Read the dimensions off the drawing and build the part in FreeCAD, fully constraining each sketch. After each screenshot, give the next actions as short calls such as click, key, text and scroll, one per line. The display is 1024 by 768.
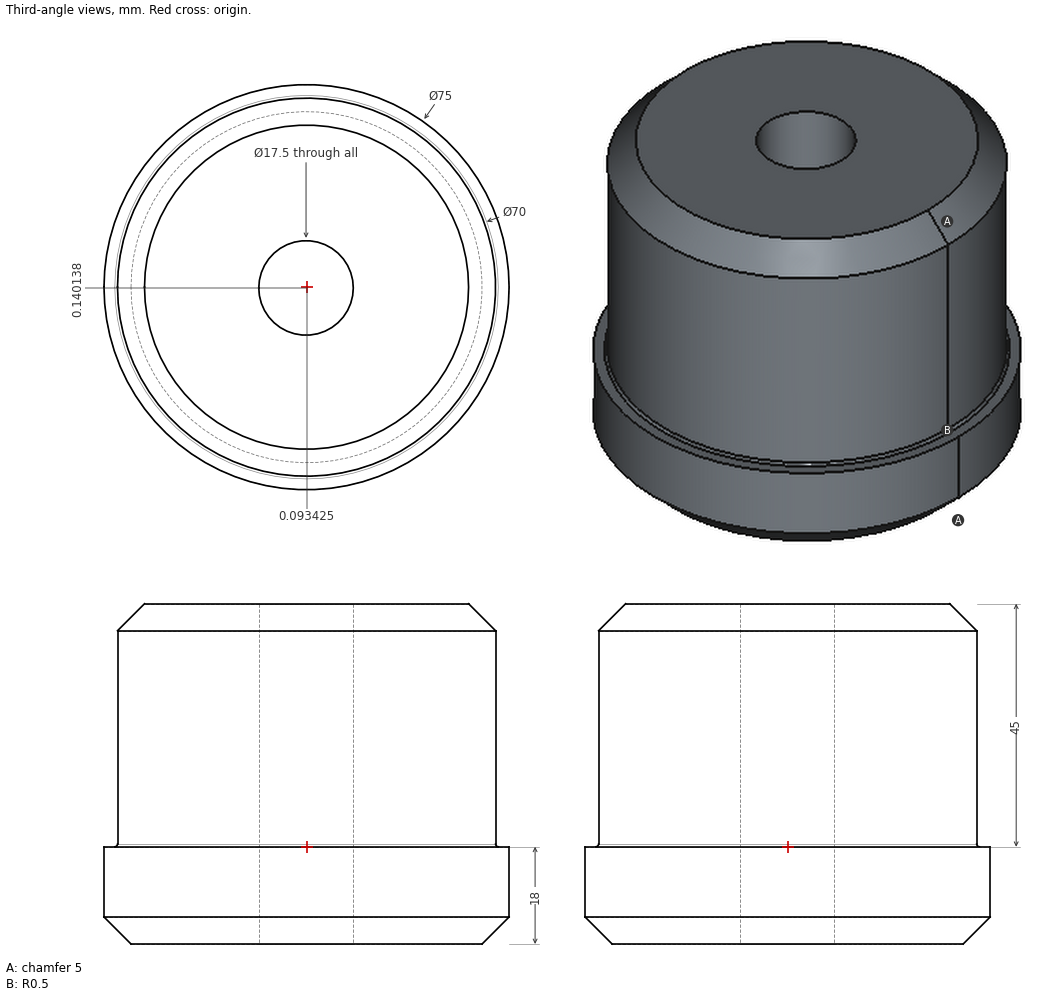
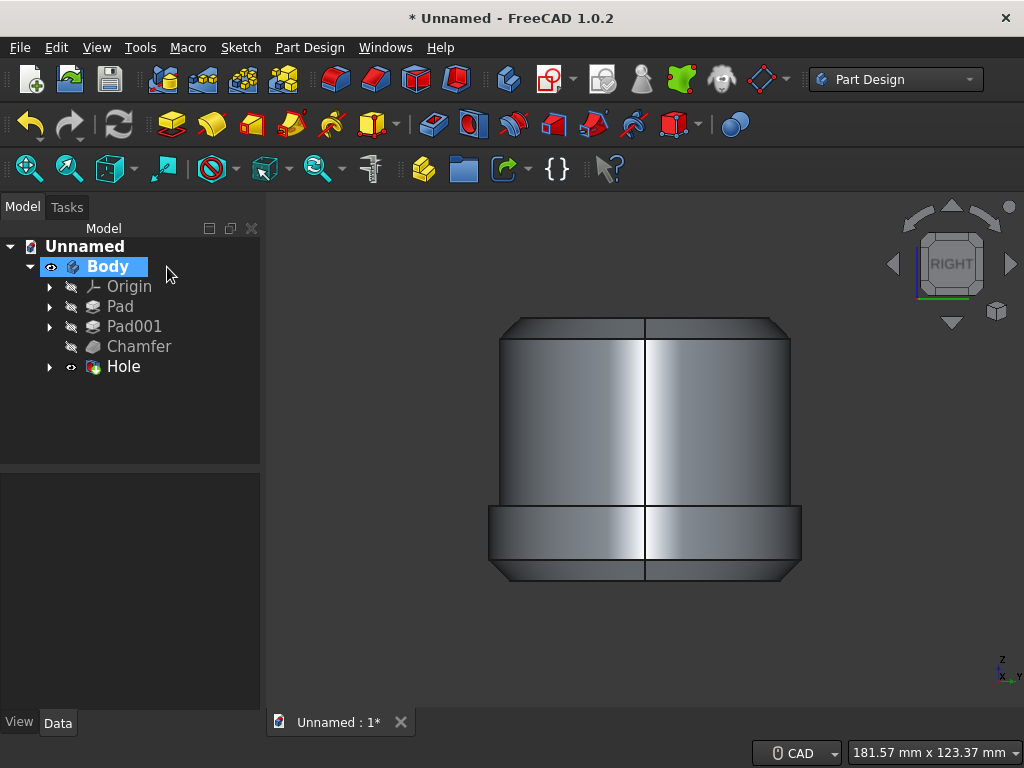
key(5)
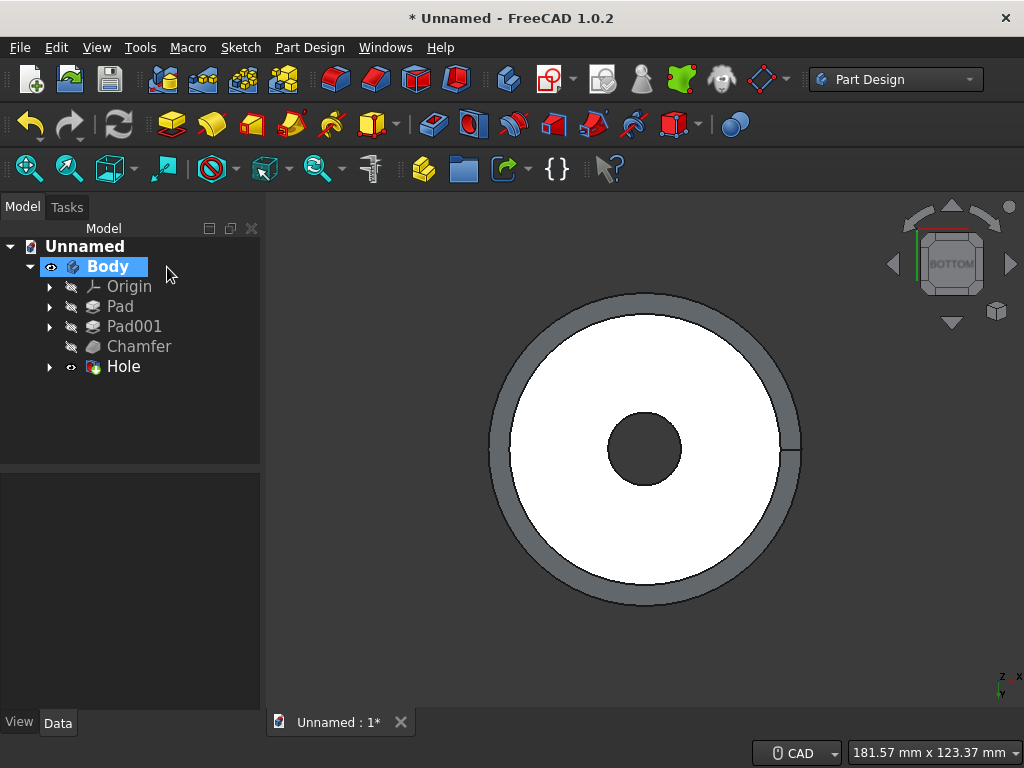
key(4)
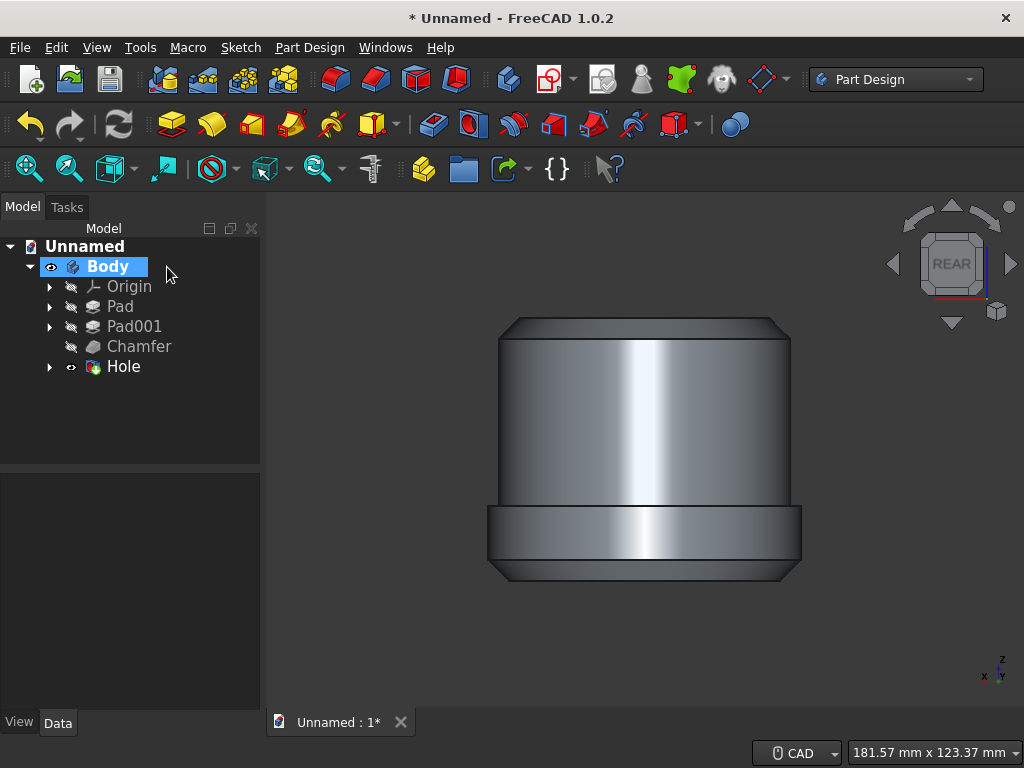
key(6)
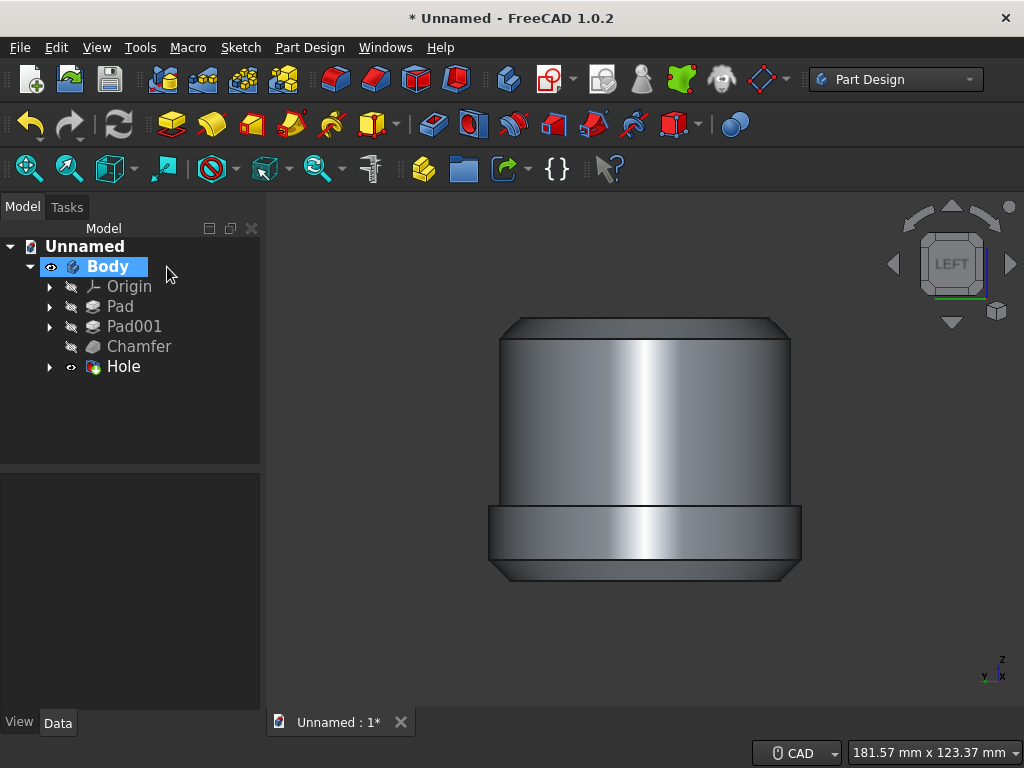
key(v)
key(3)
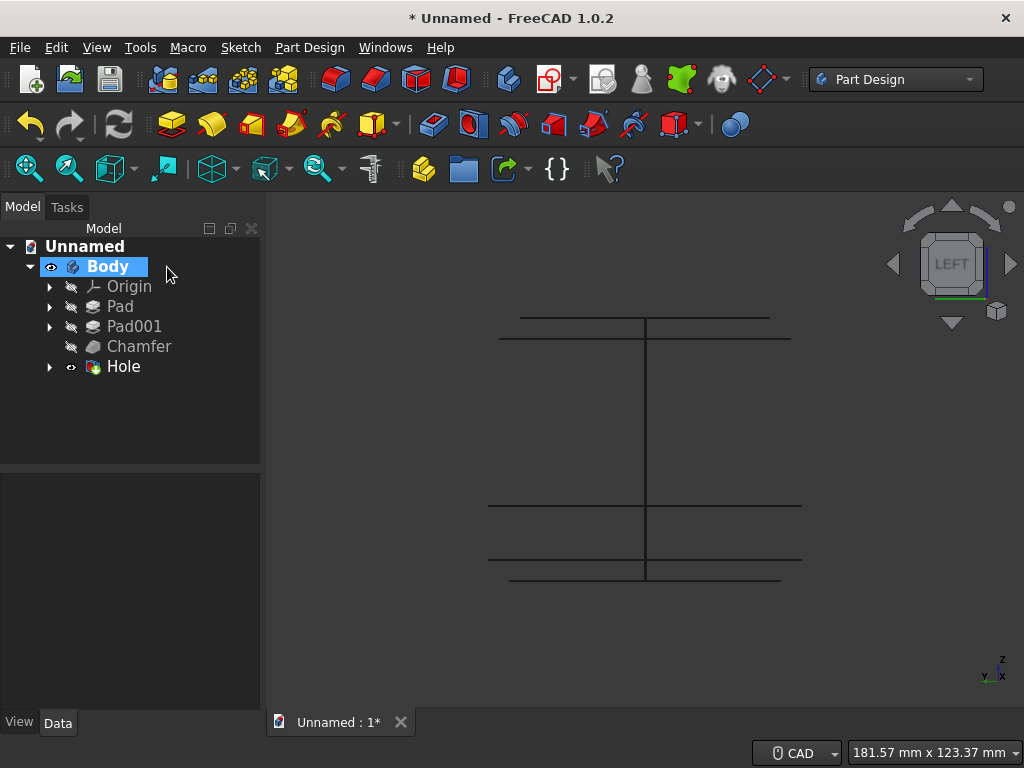
key(0)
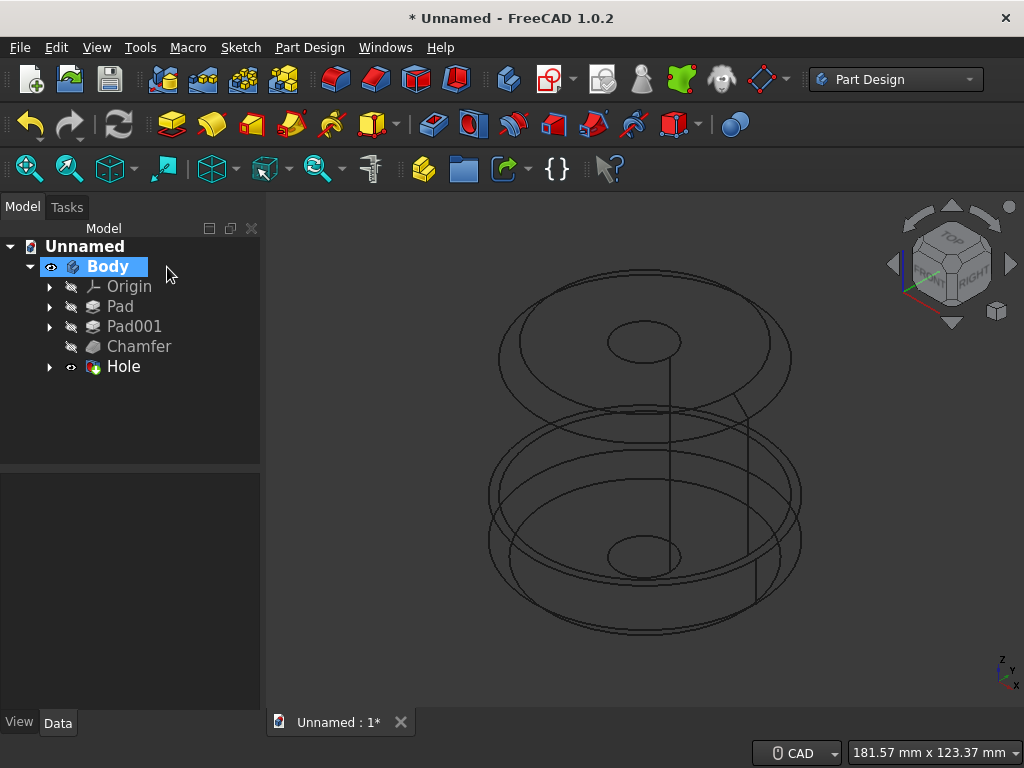
click(542, 435)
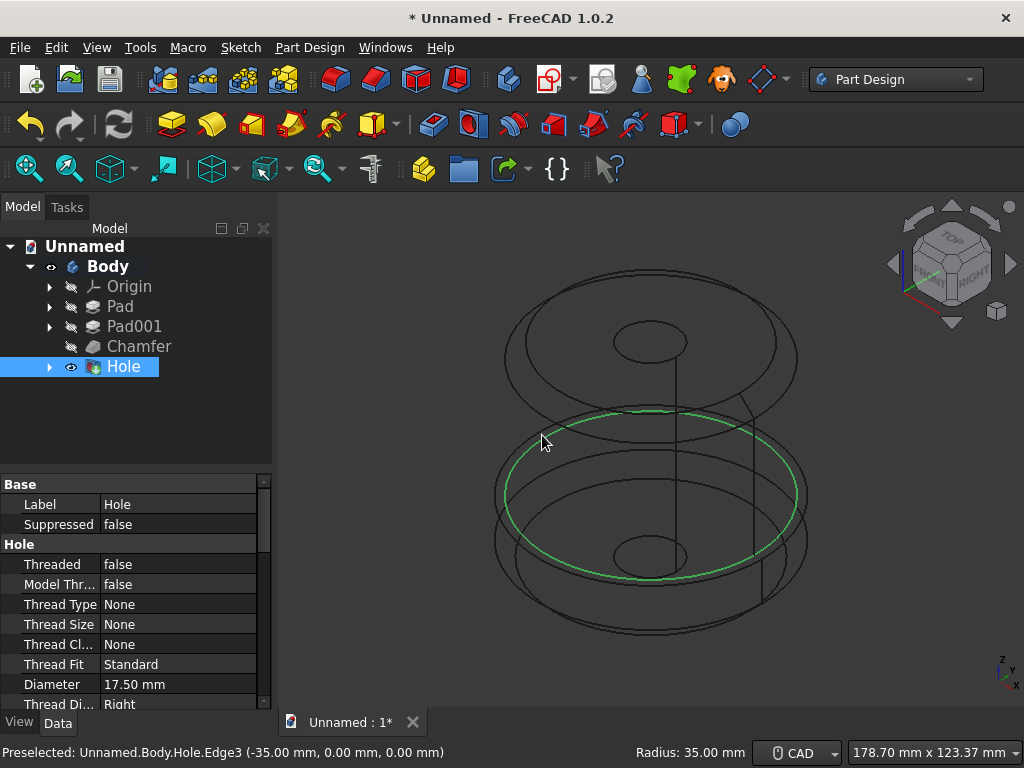
key(v)
key(1)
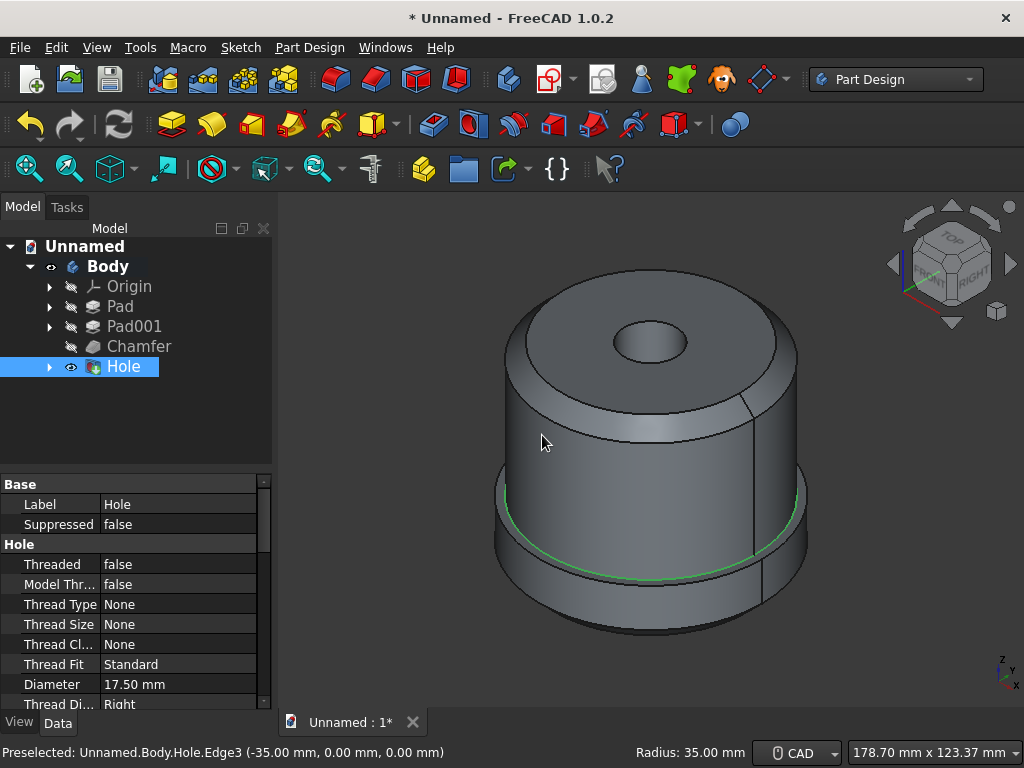
click(336, 80)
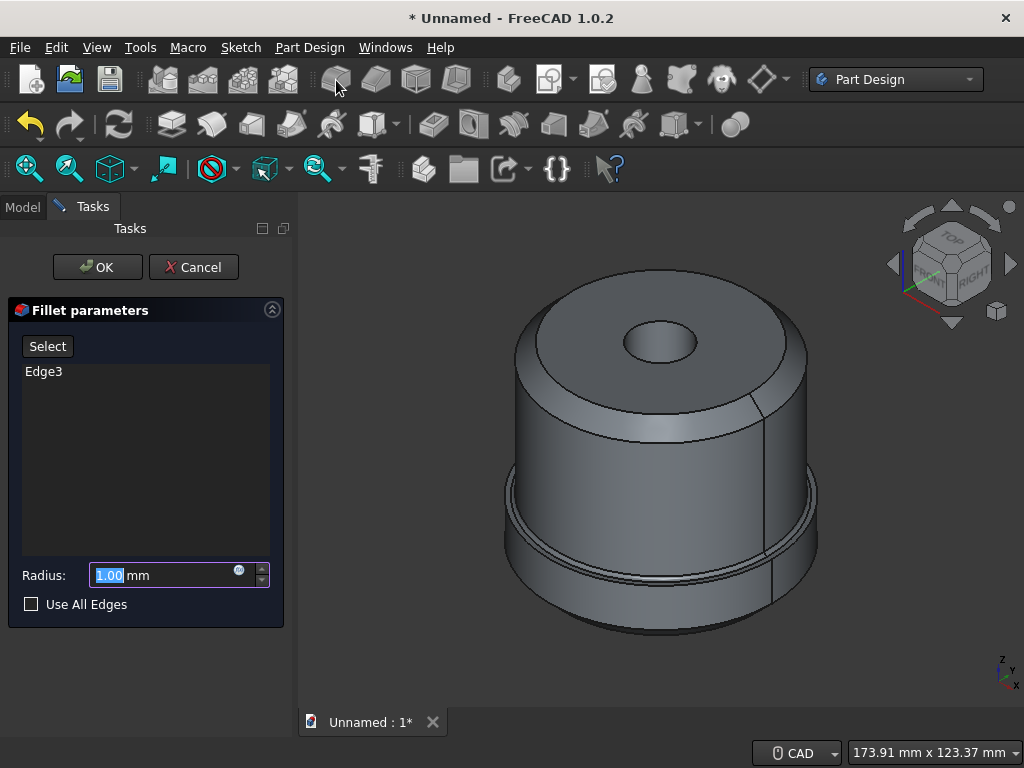
text(0.5)
key(Tab)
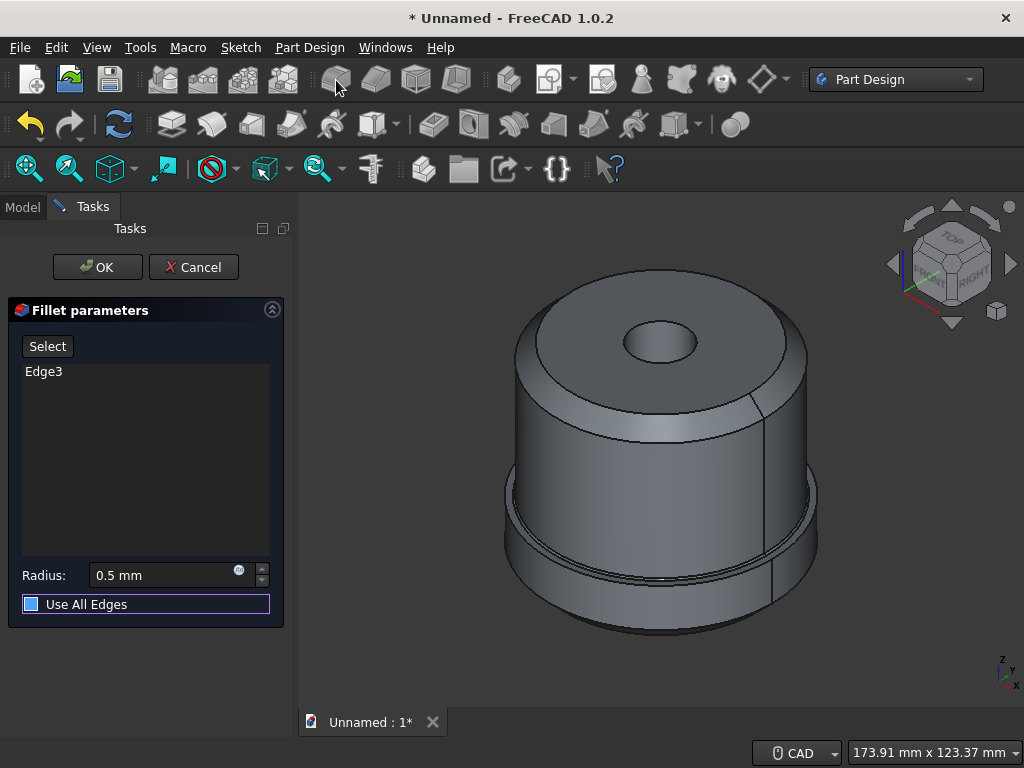
click(98, 267)